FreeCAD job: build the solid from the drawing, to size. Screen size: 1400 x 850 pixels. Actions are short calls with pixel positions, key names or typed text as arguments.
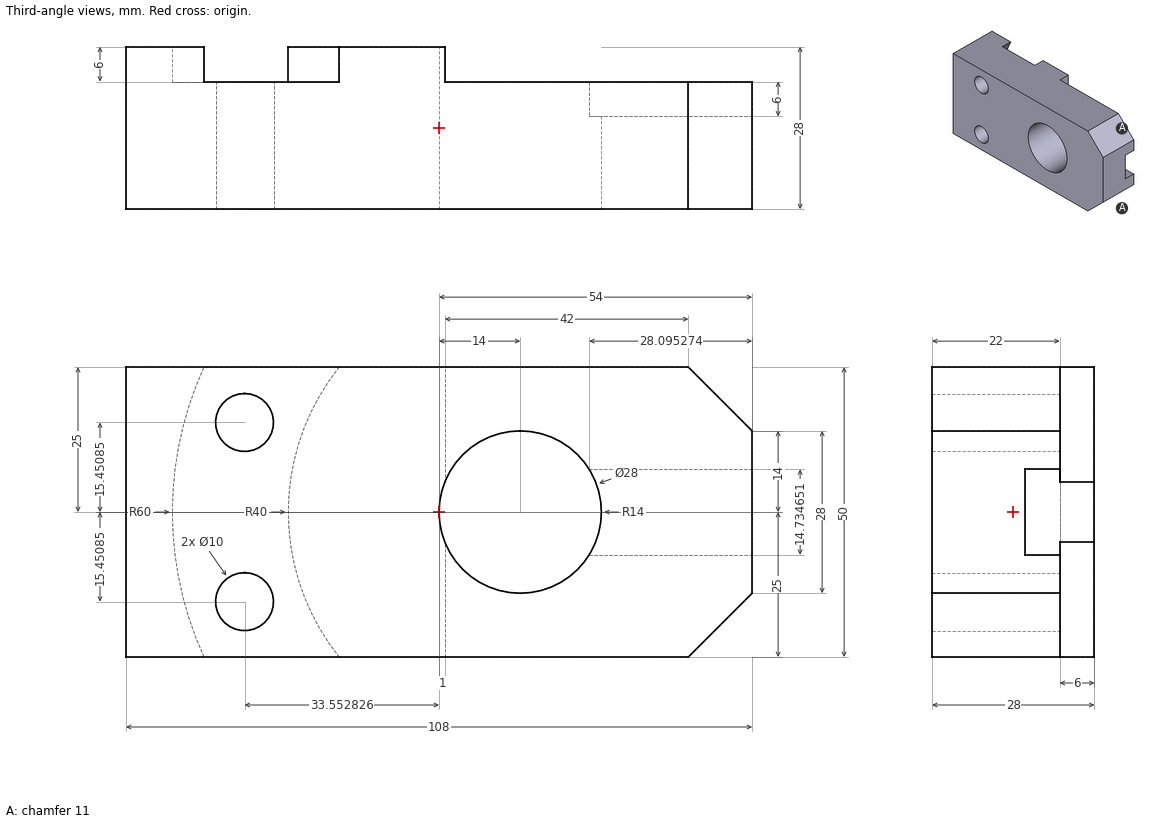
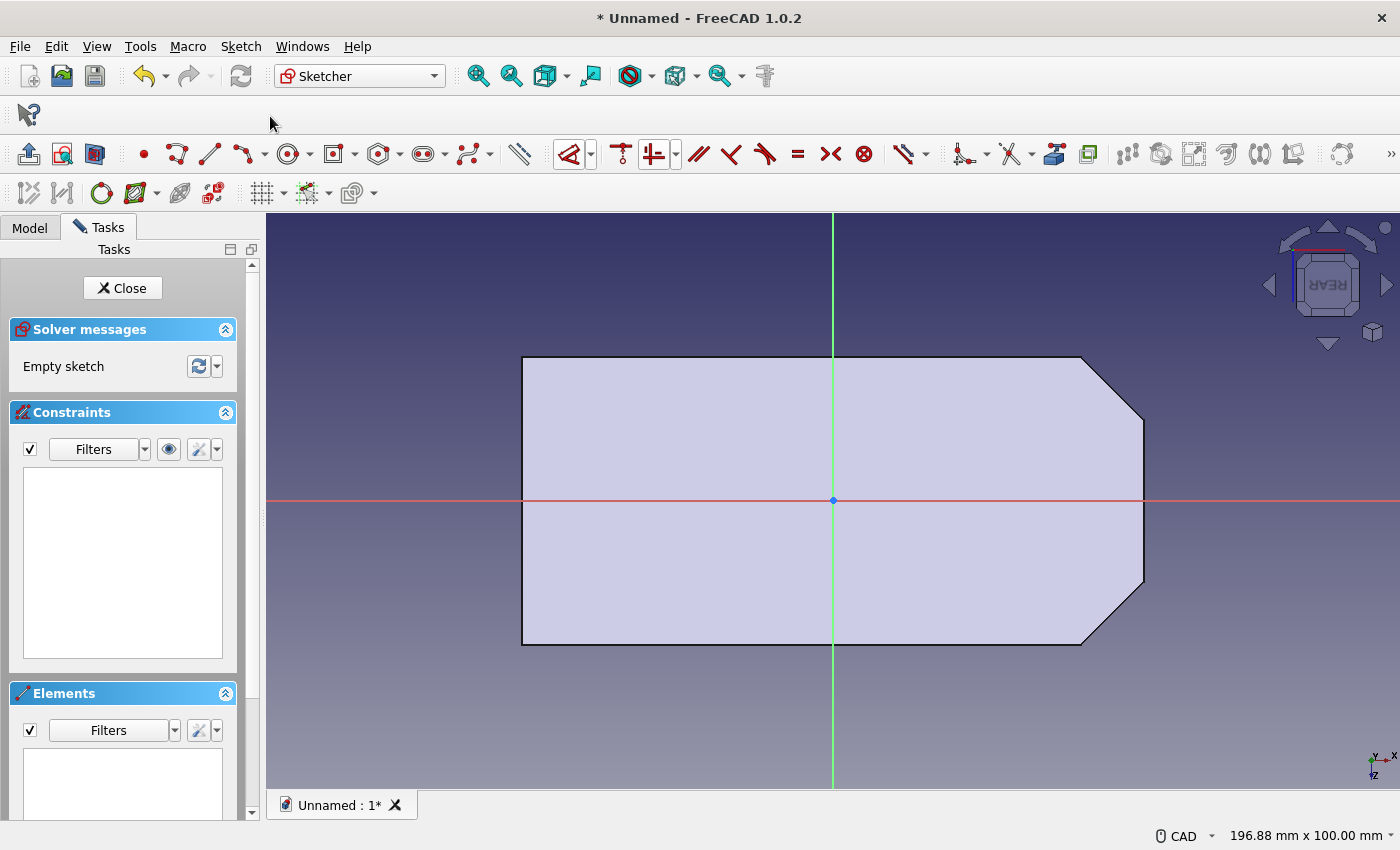
scroll(1035, 501, up, 4)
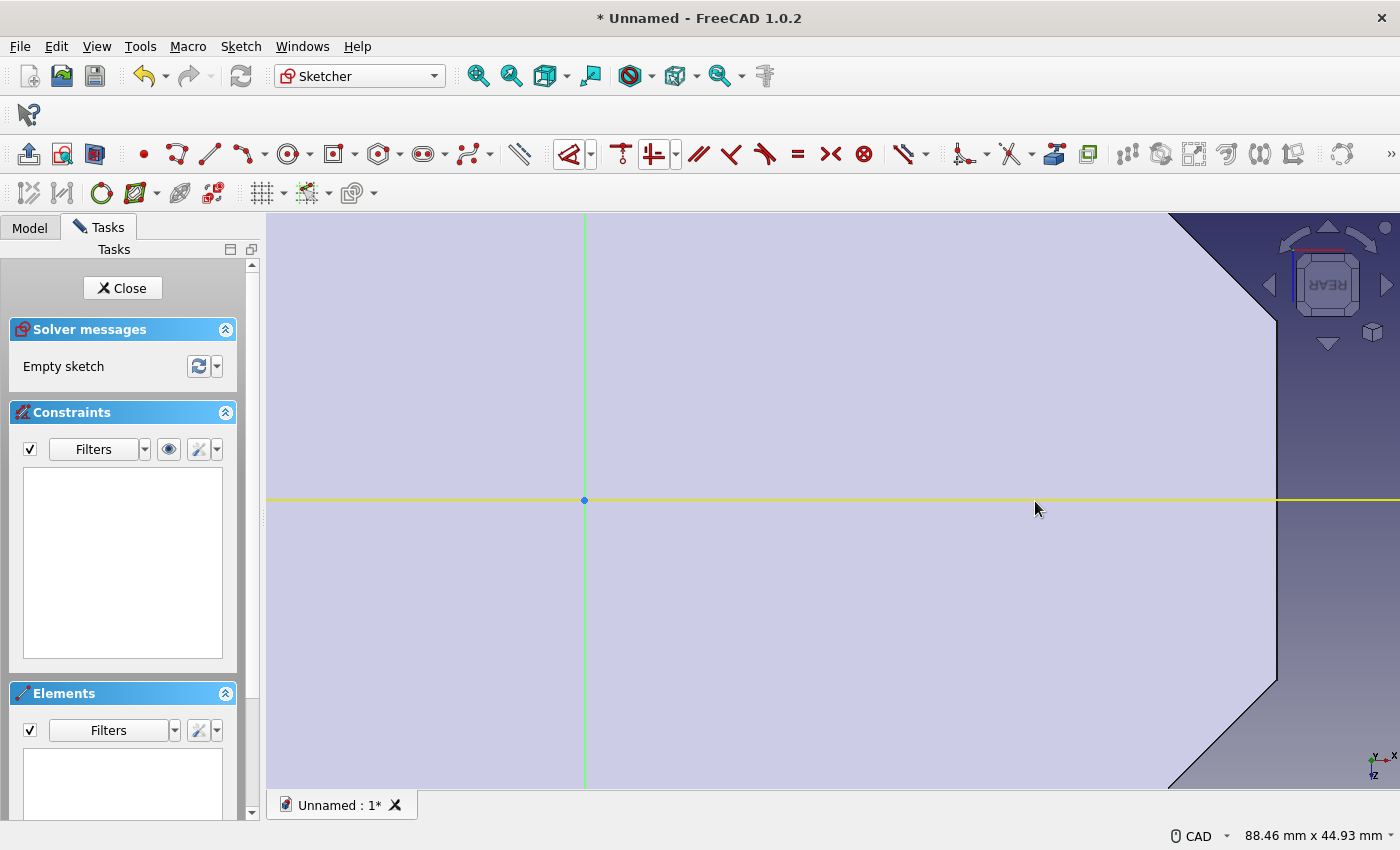
click(288, 154)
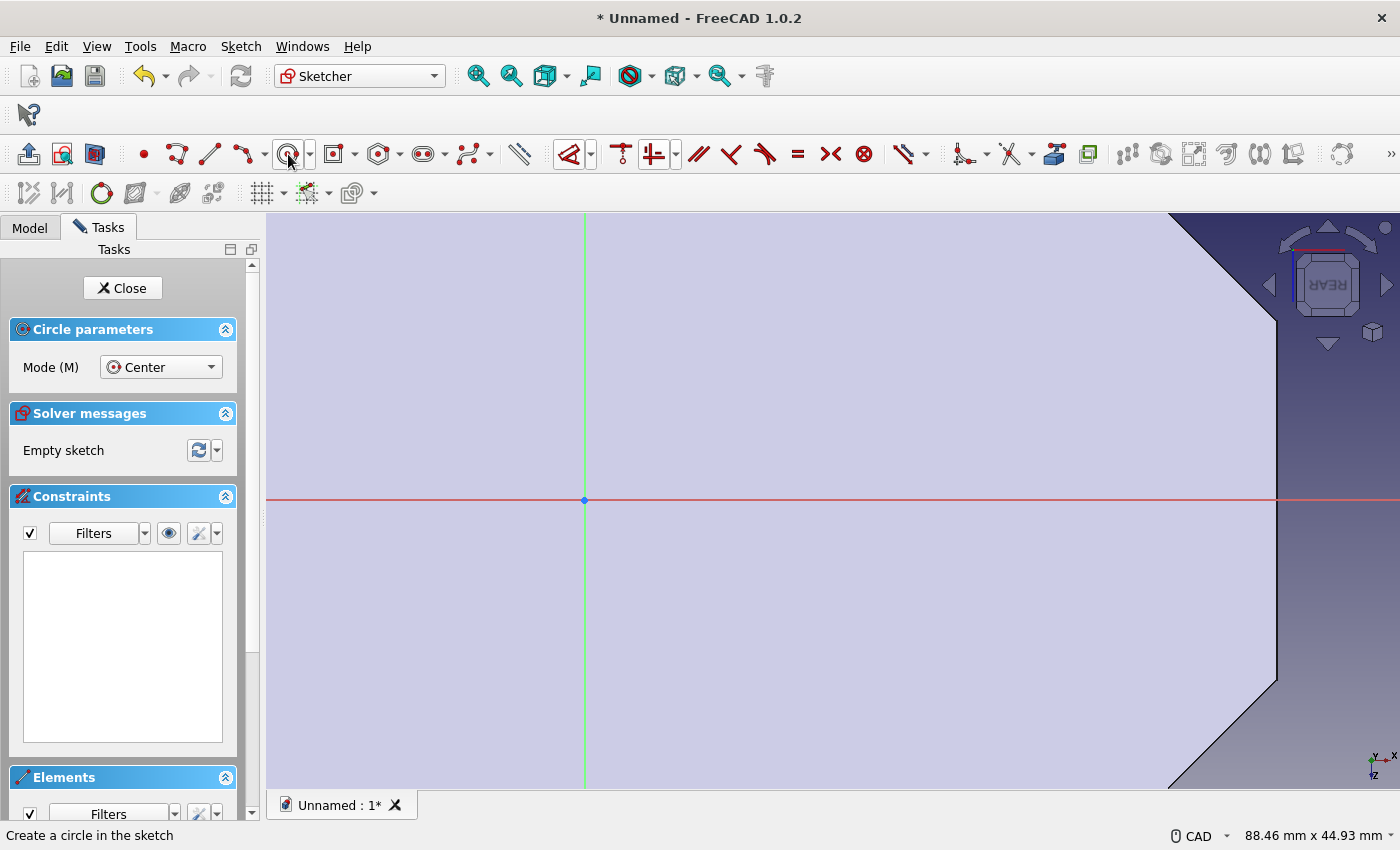
click(764, 500)
move(891, 373)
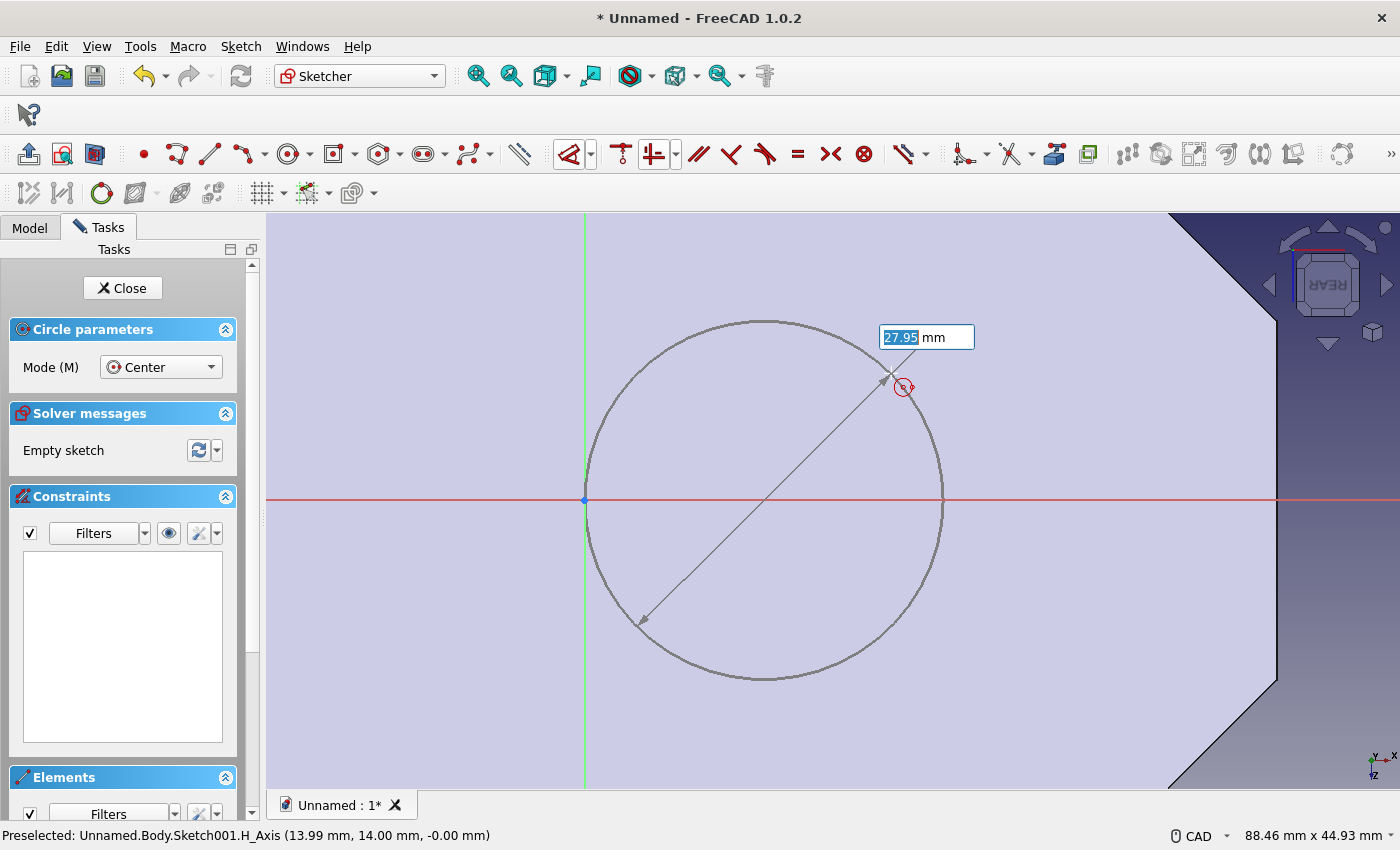
text(28)
key(Return)
key(Escape)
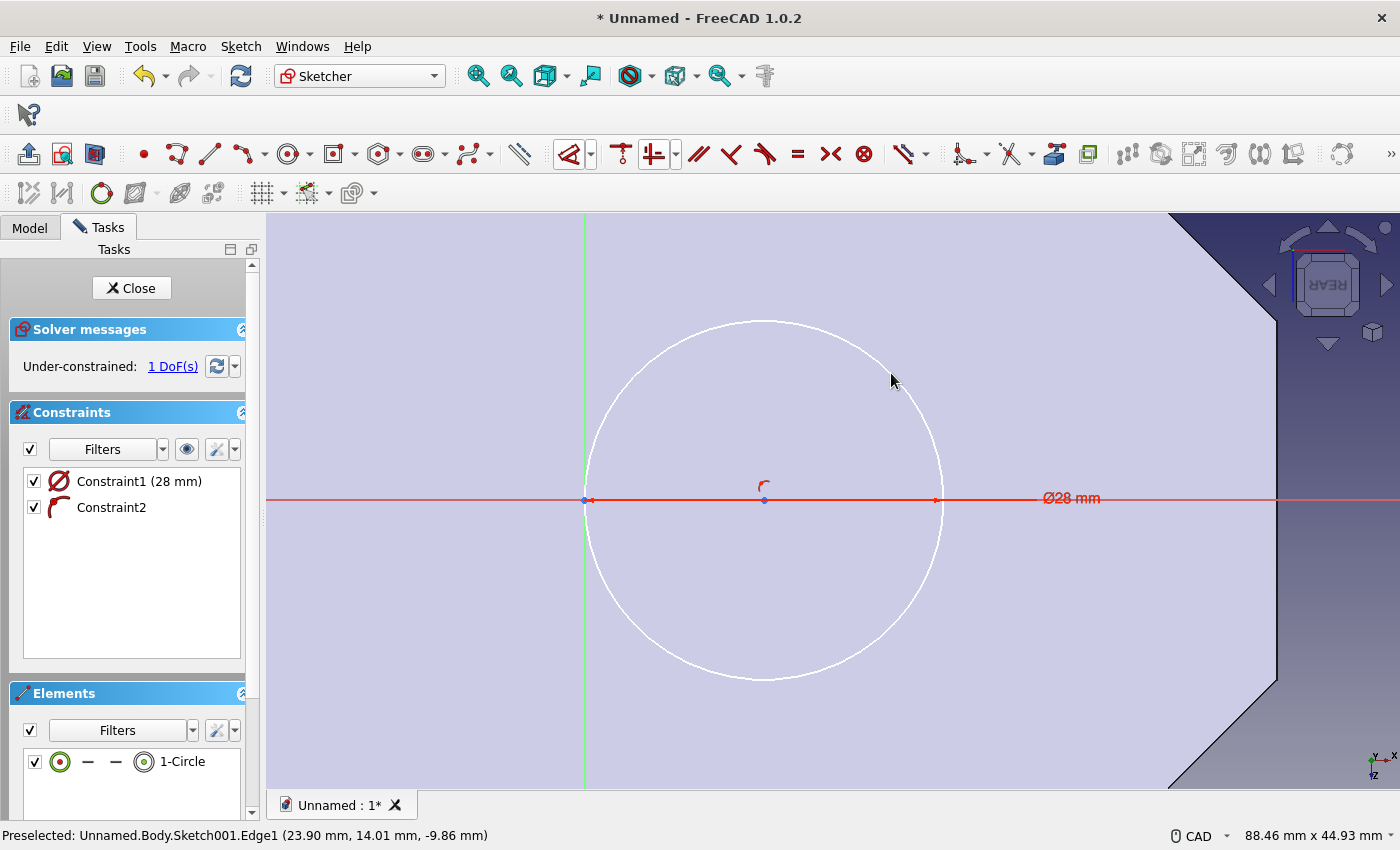
click(568, 154)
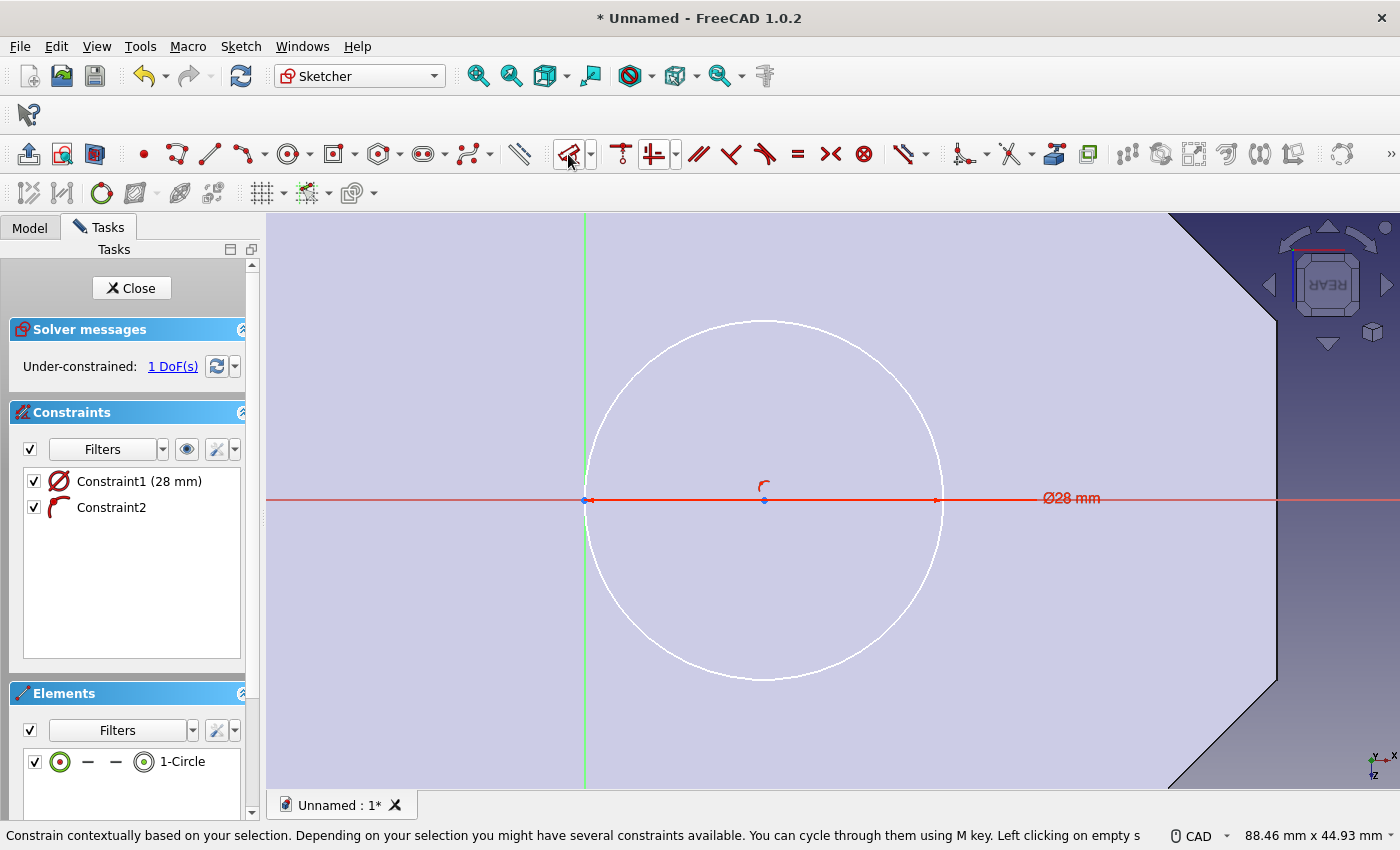
click(764, 500)
click(674, 534)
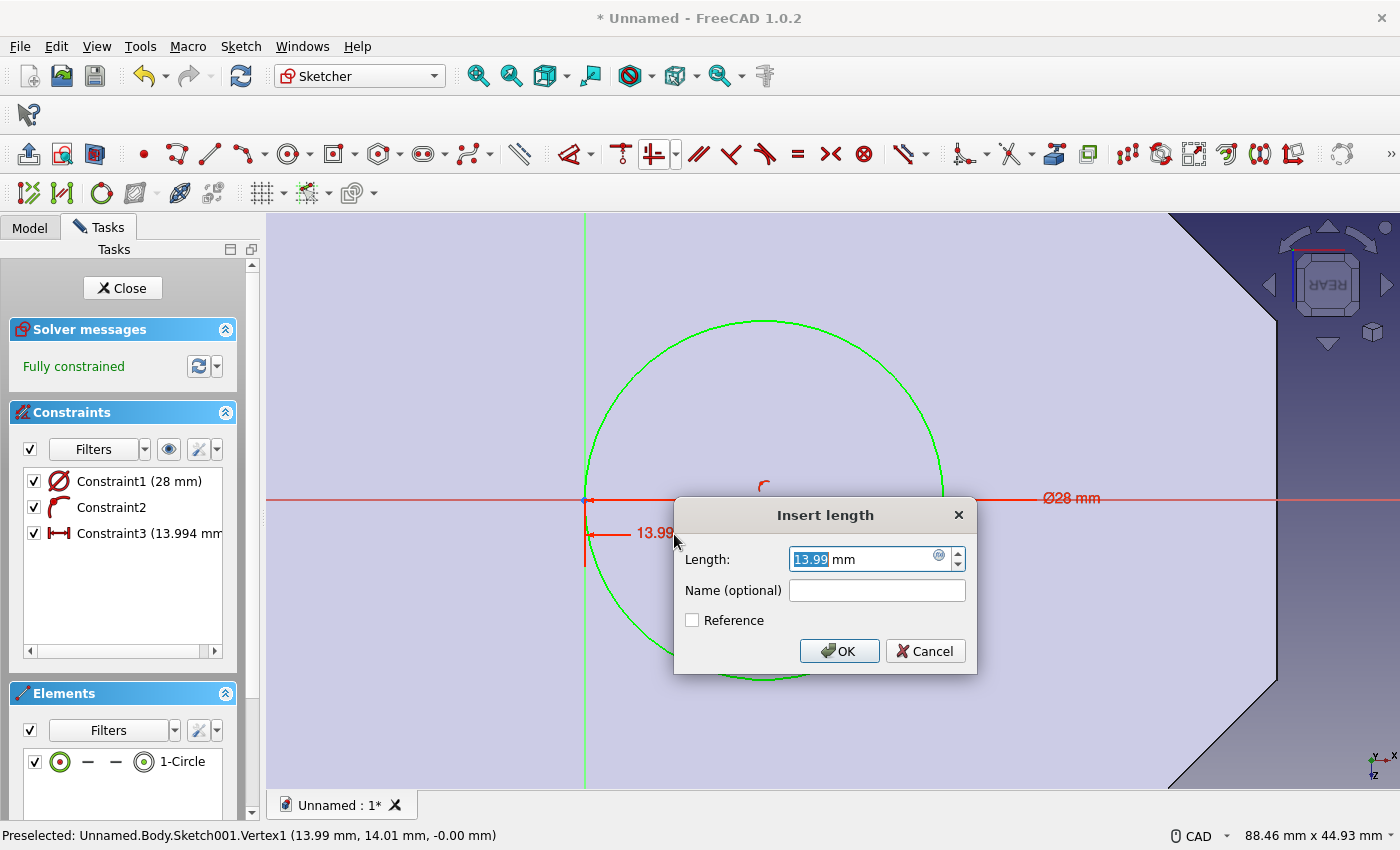
text(14)
key(Return)
key(Escape)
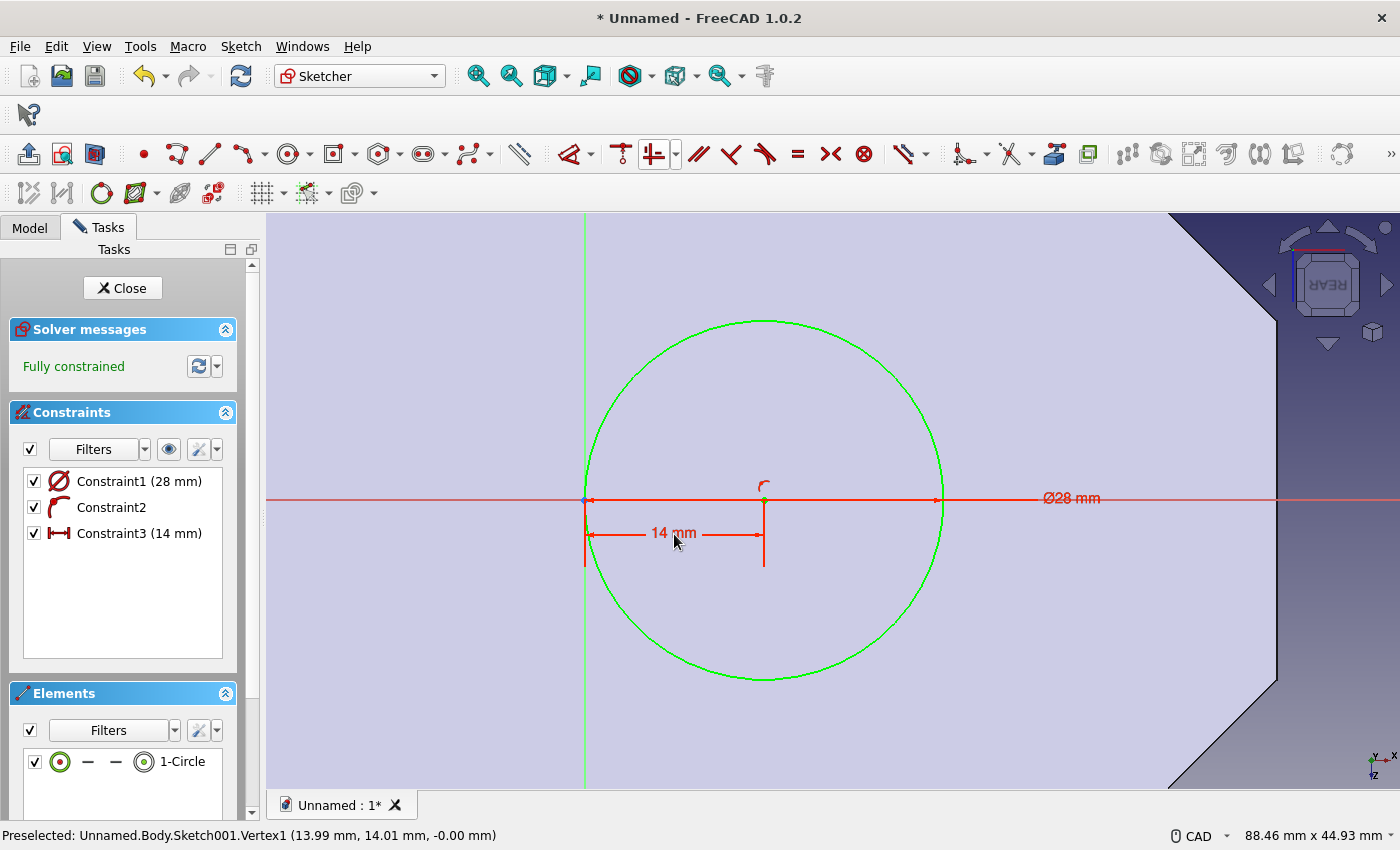
click(123, 288)